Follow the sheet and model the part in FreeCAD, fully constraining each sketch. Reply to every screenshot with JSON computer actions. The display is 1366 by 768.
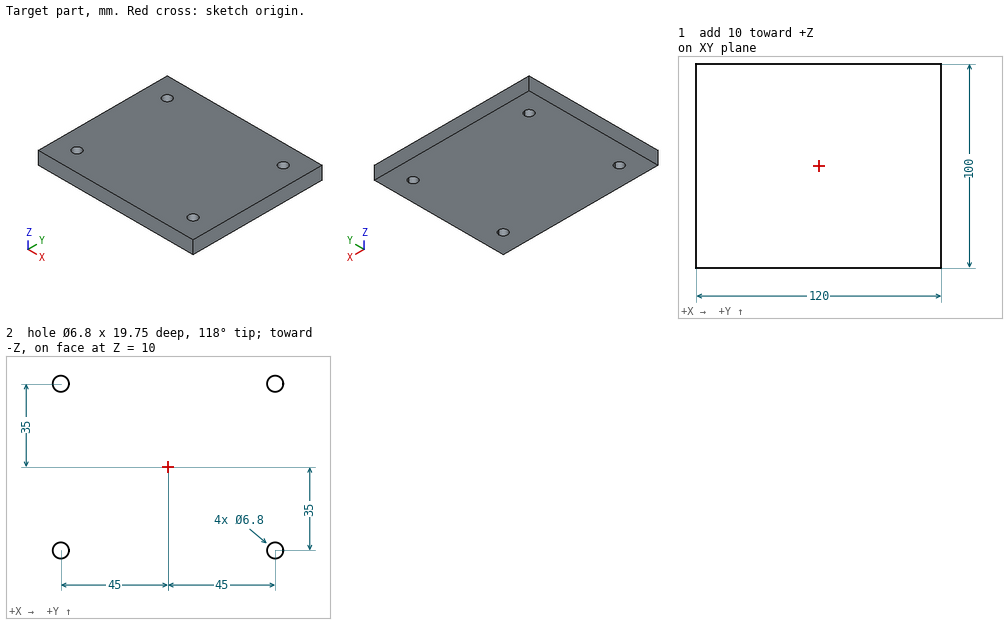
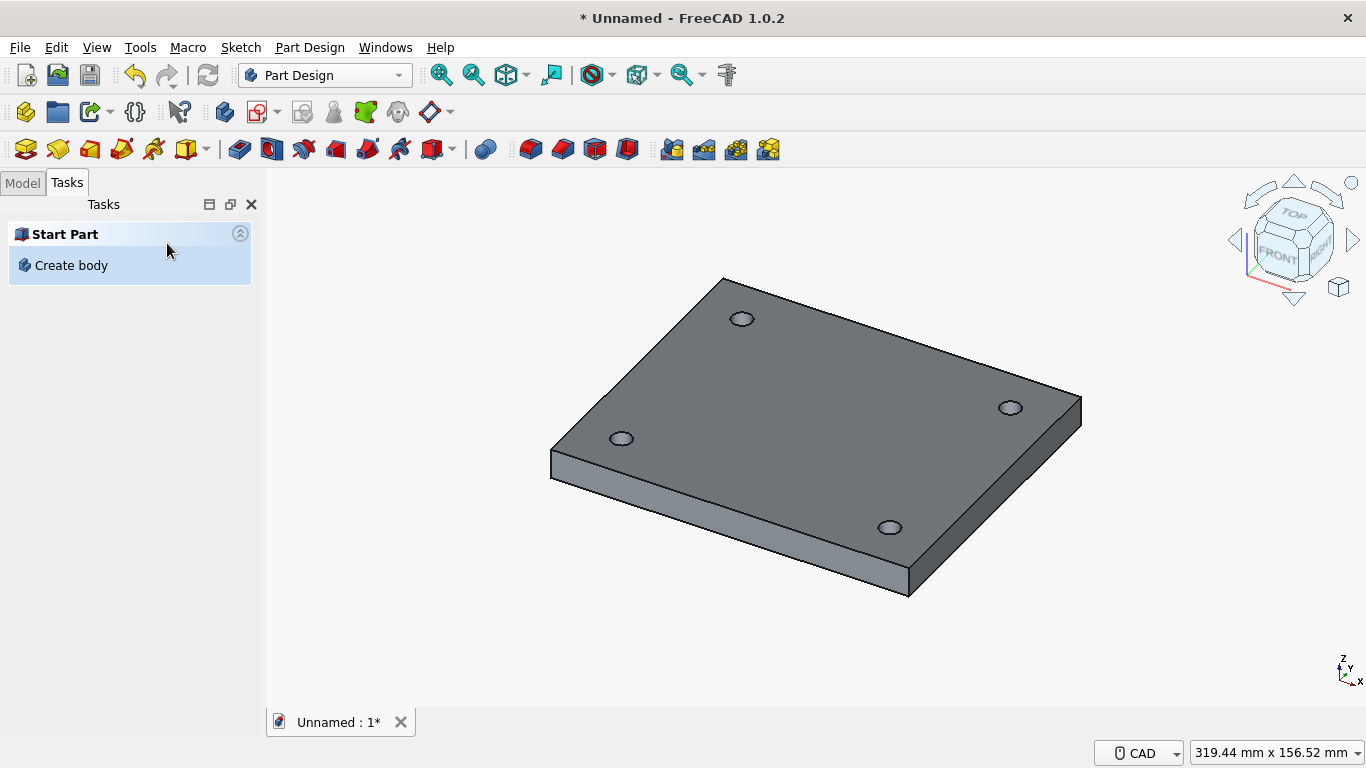
{"action": "key", "text": "0"}